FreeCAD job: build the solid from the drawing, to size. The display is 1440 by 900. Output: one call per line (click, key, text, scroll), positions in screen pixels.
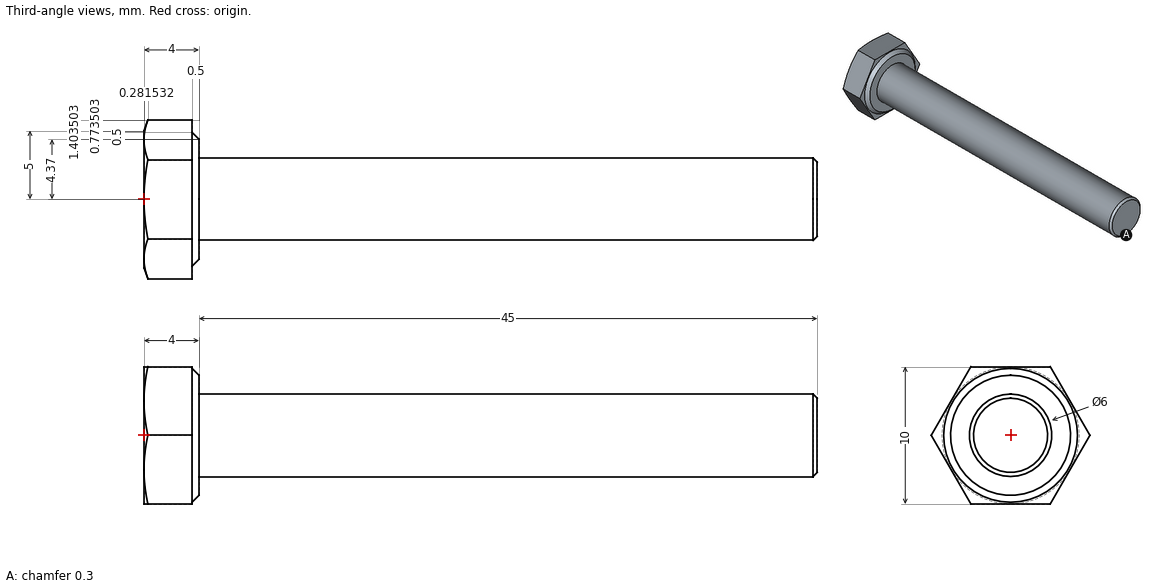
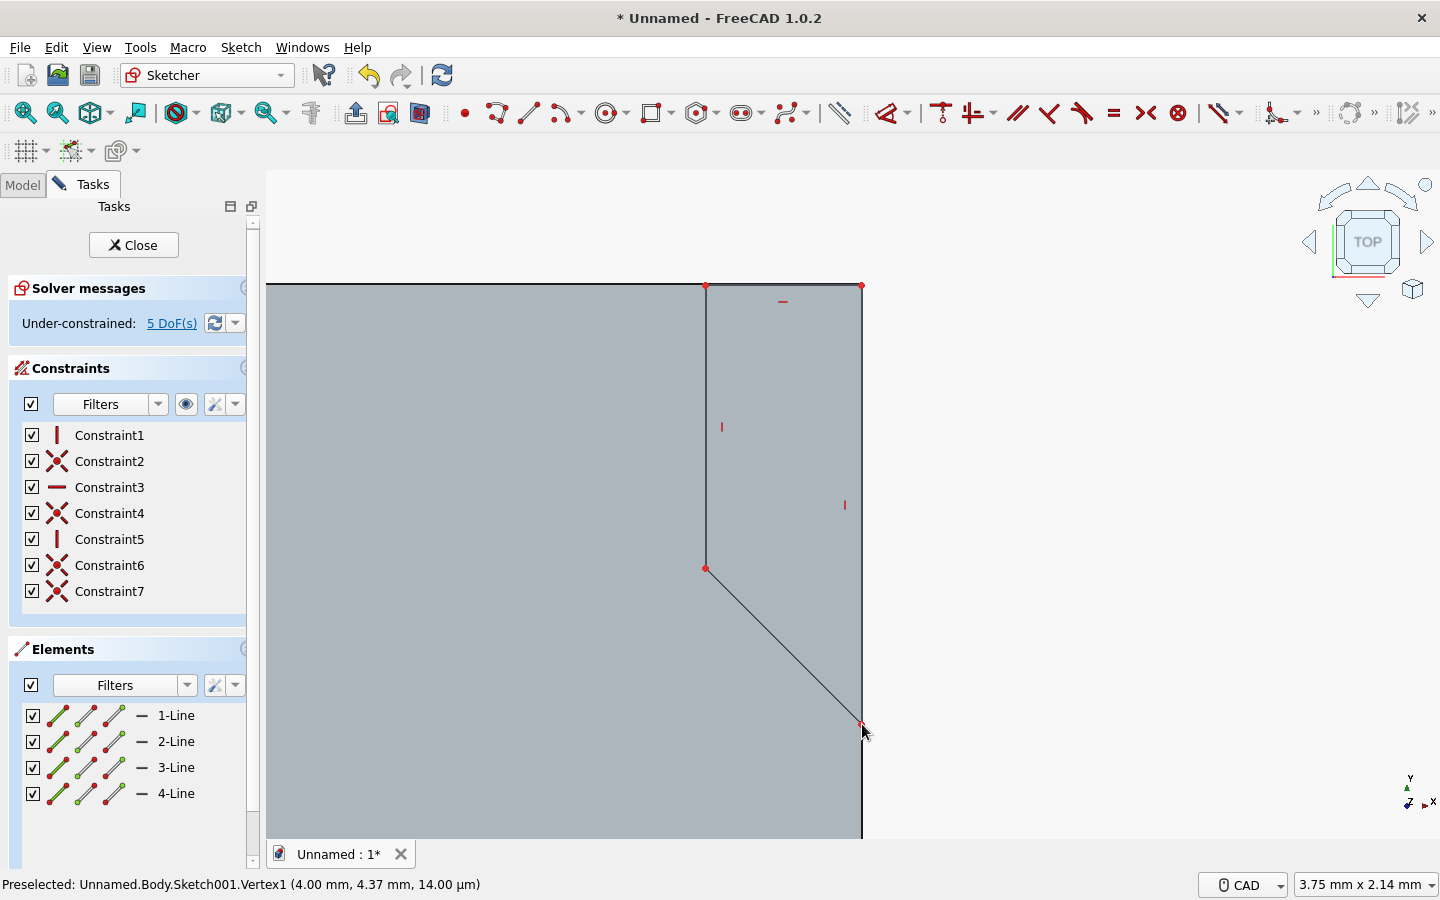
click(886, 114)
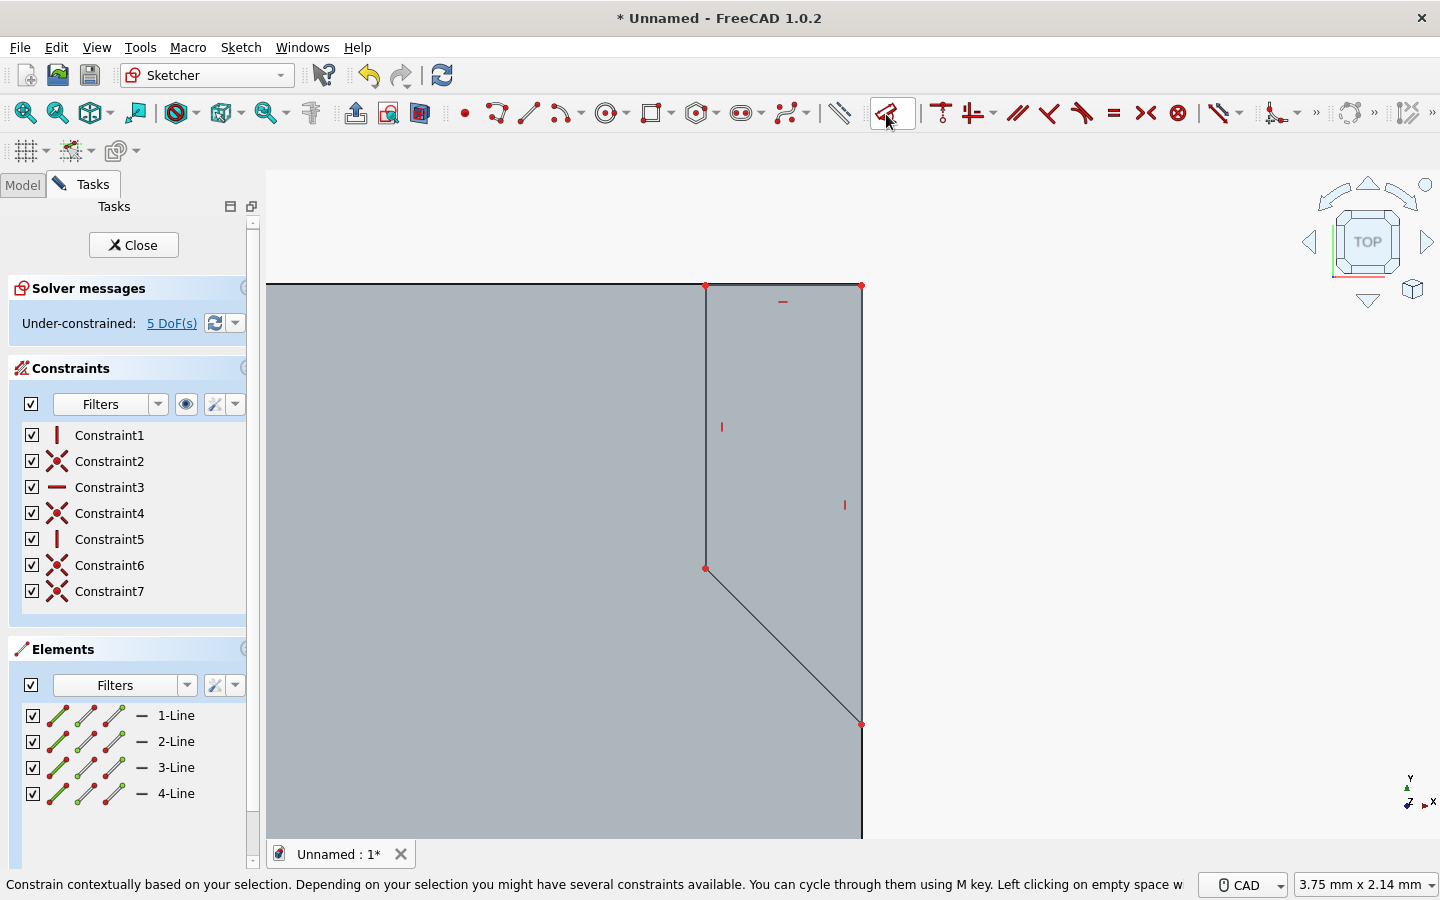
click(862, 724)
click(578, 690)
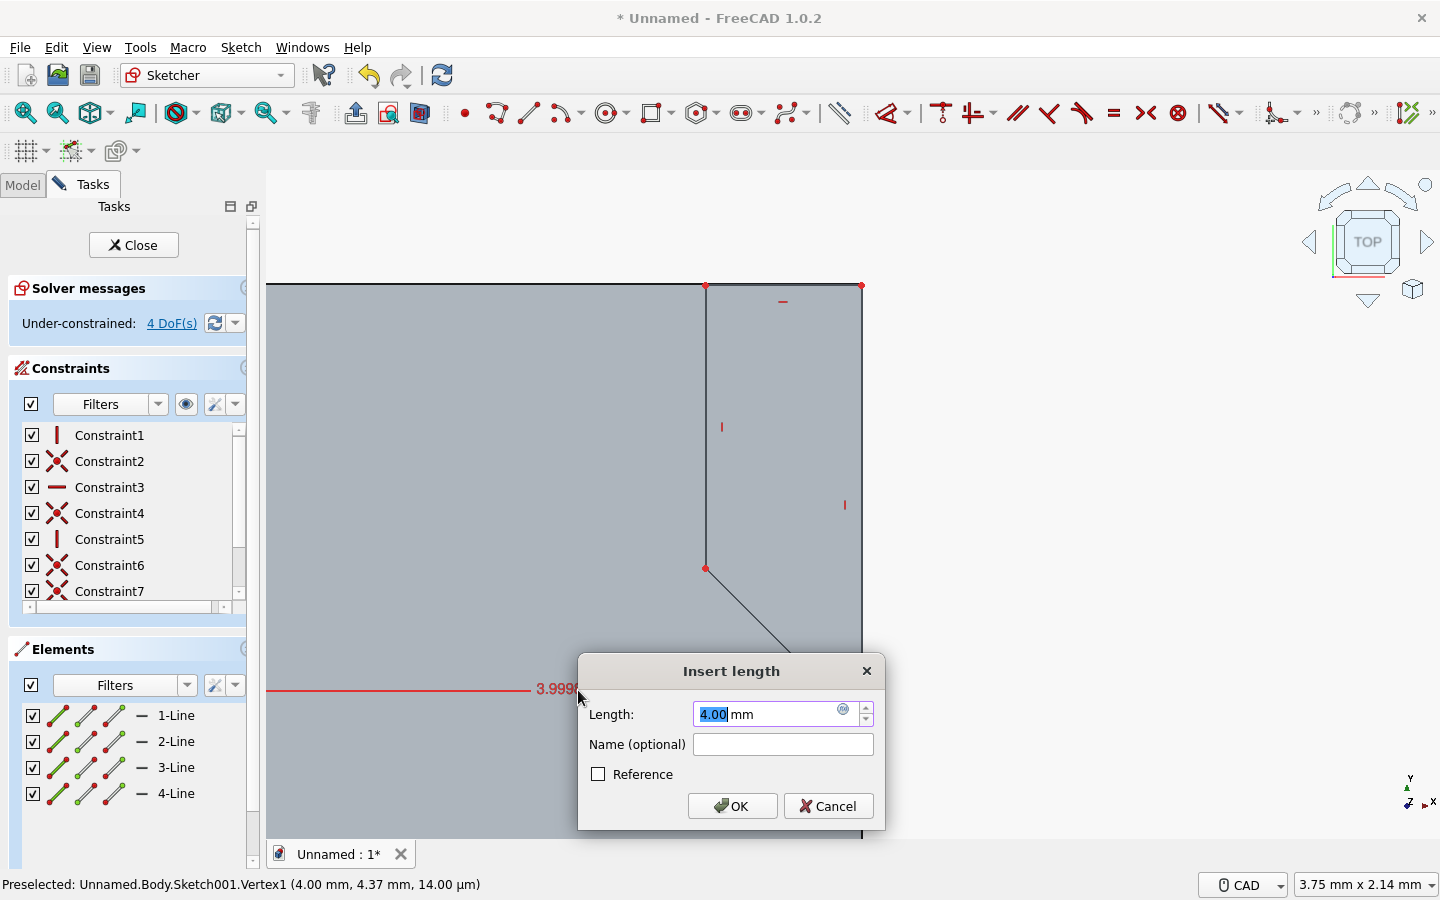
text(4)
key(Return)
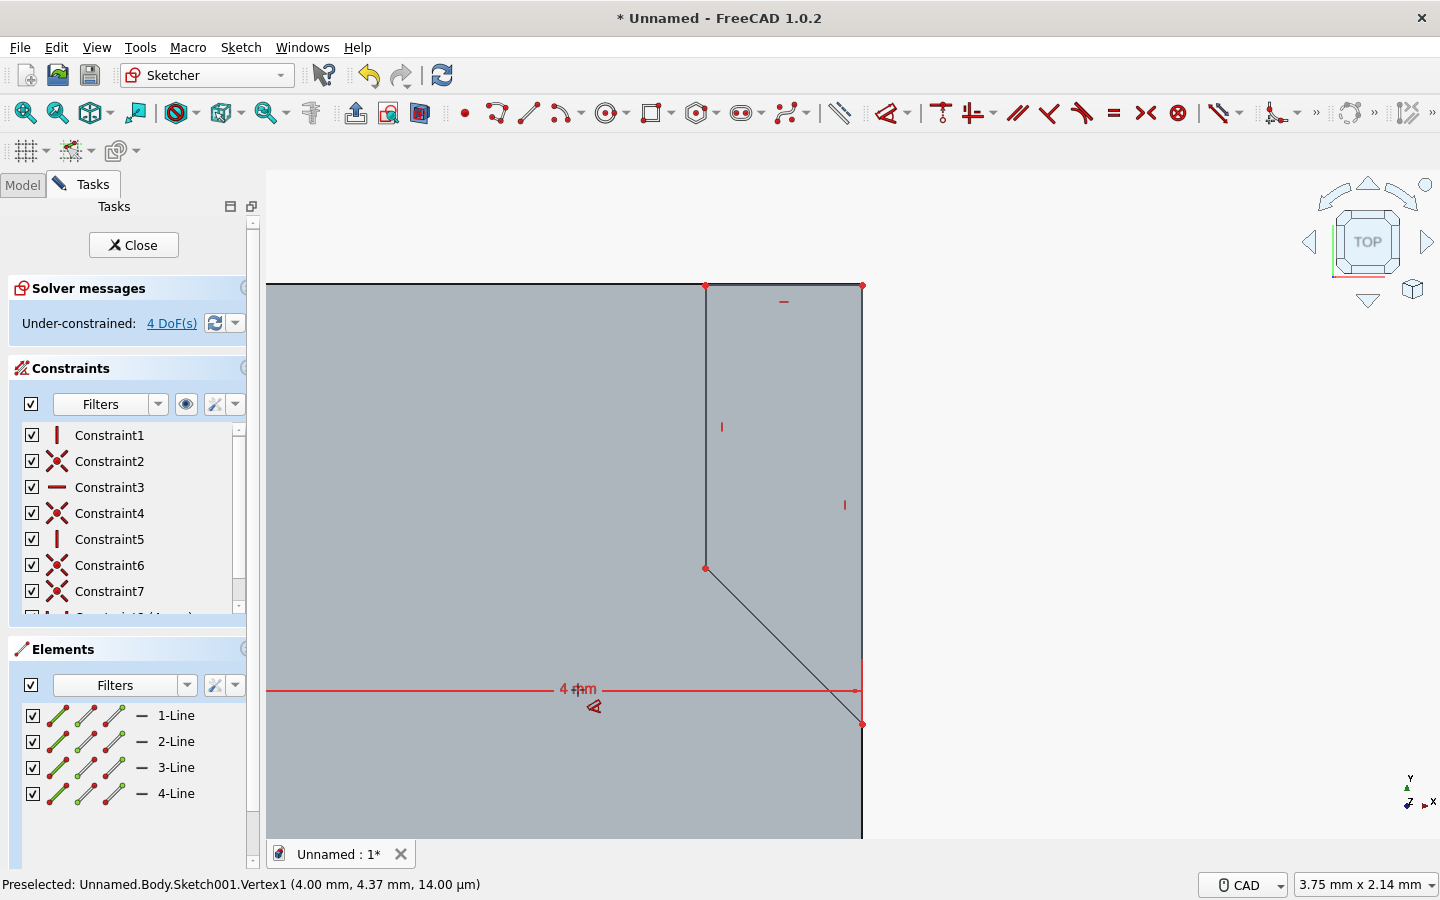
click(815, 285)
click(784, 251)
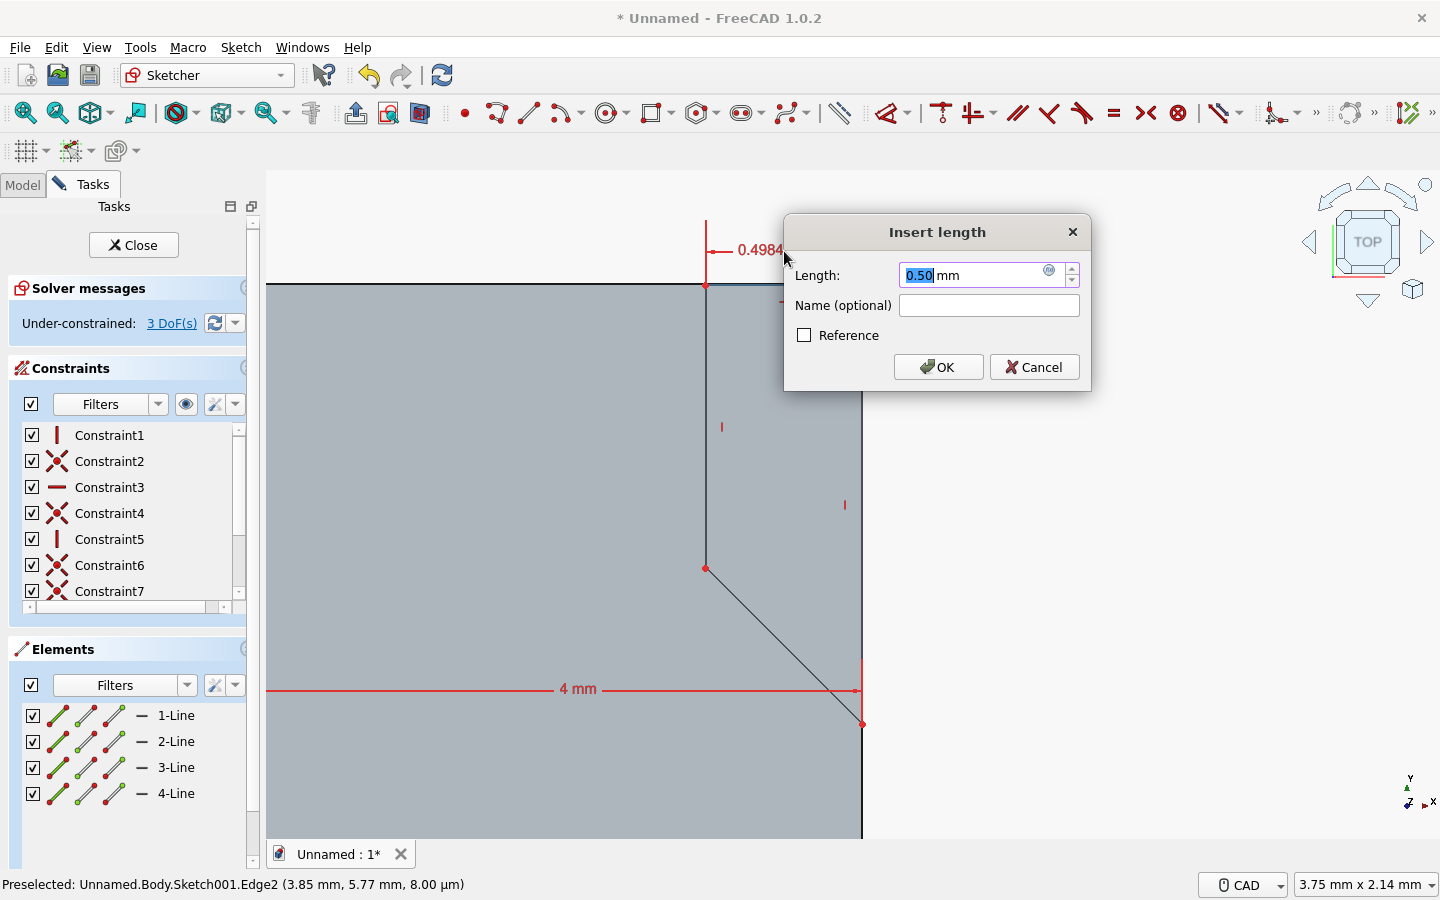
text(0.5)
key(Return)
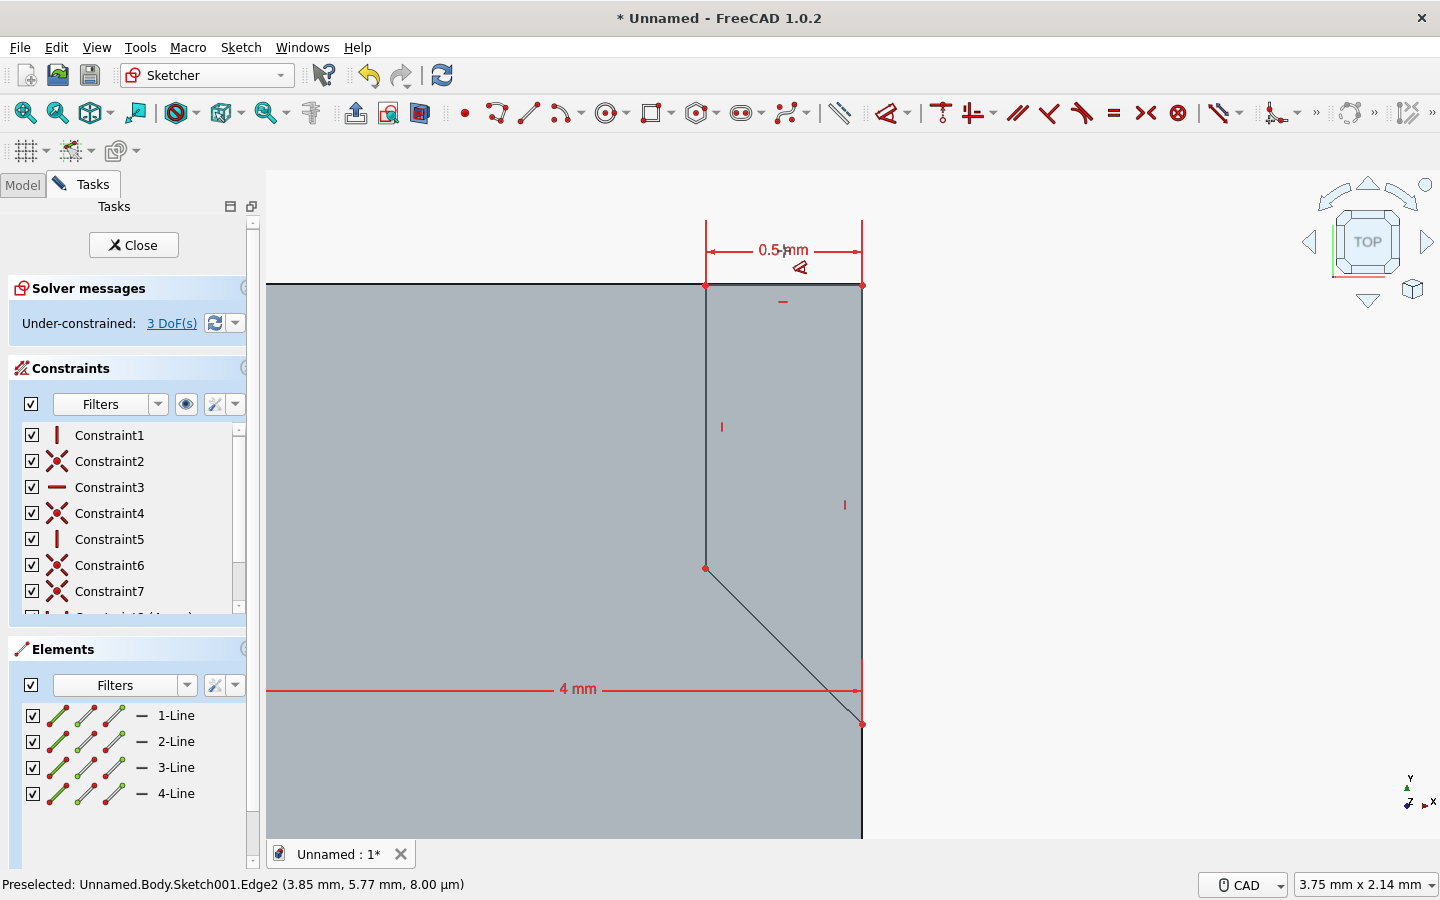
click(752, 615)
click(672, 646)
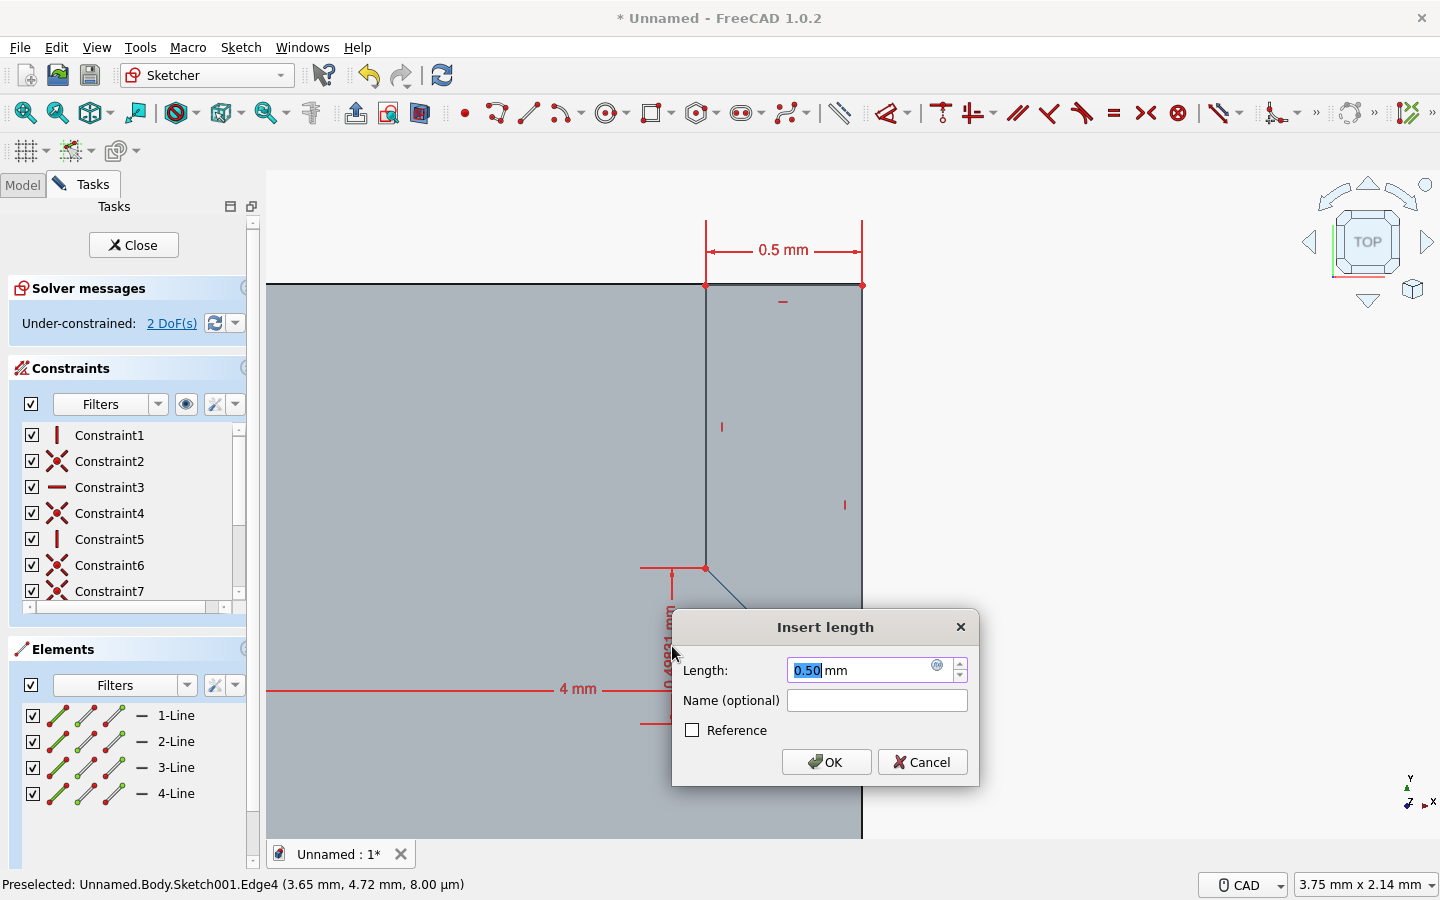
text(0.5)
key(Return)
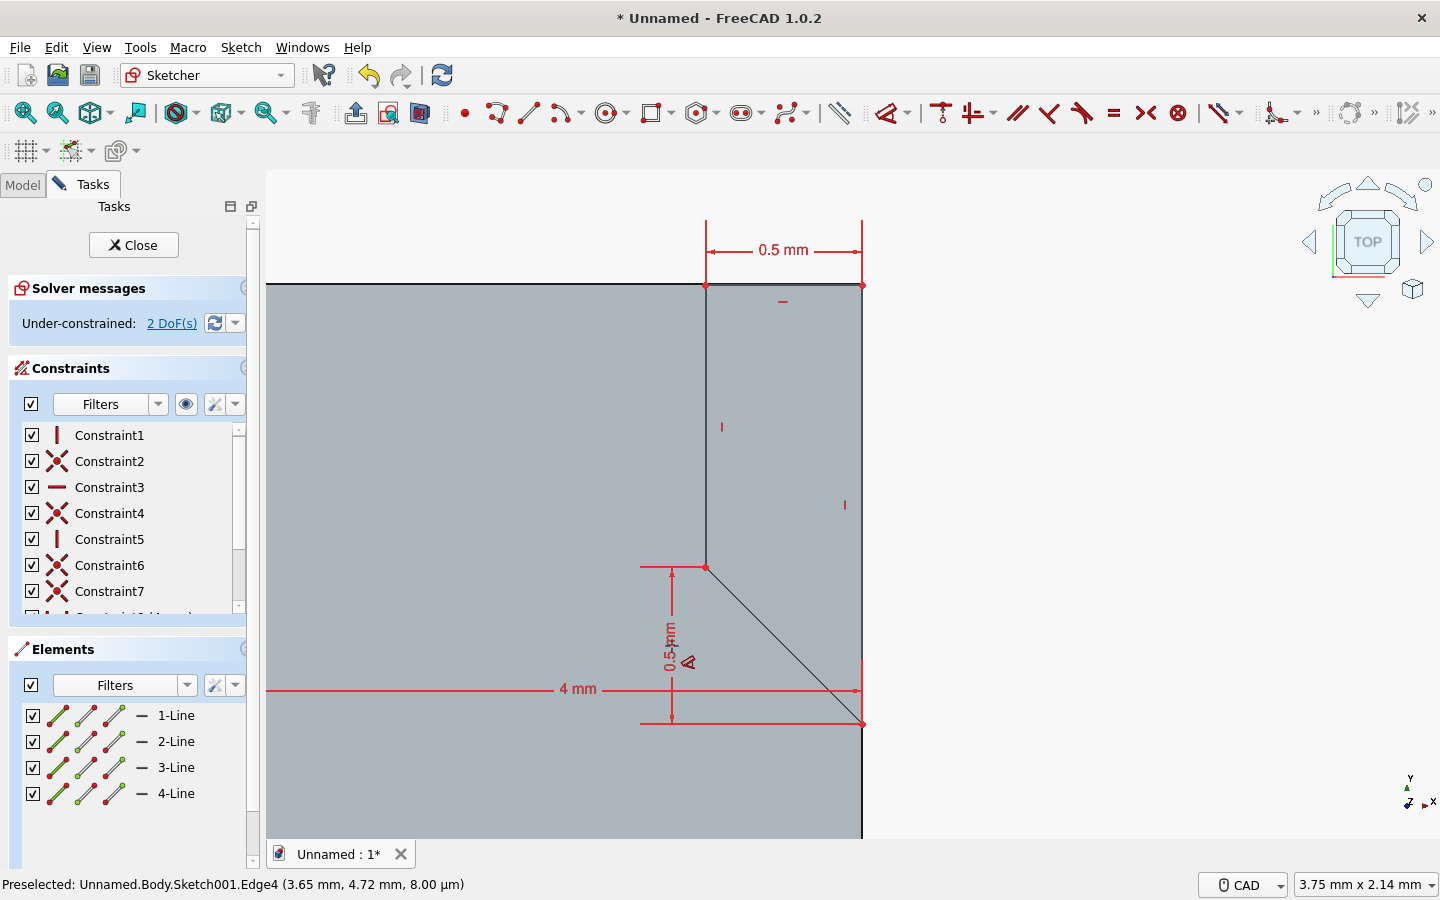
click(862, 724)
click(896, 768)